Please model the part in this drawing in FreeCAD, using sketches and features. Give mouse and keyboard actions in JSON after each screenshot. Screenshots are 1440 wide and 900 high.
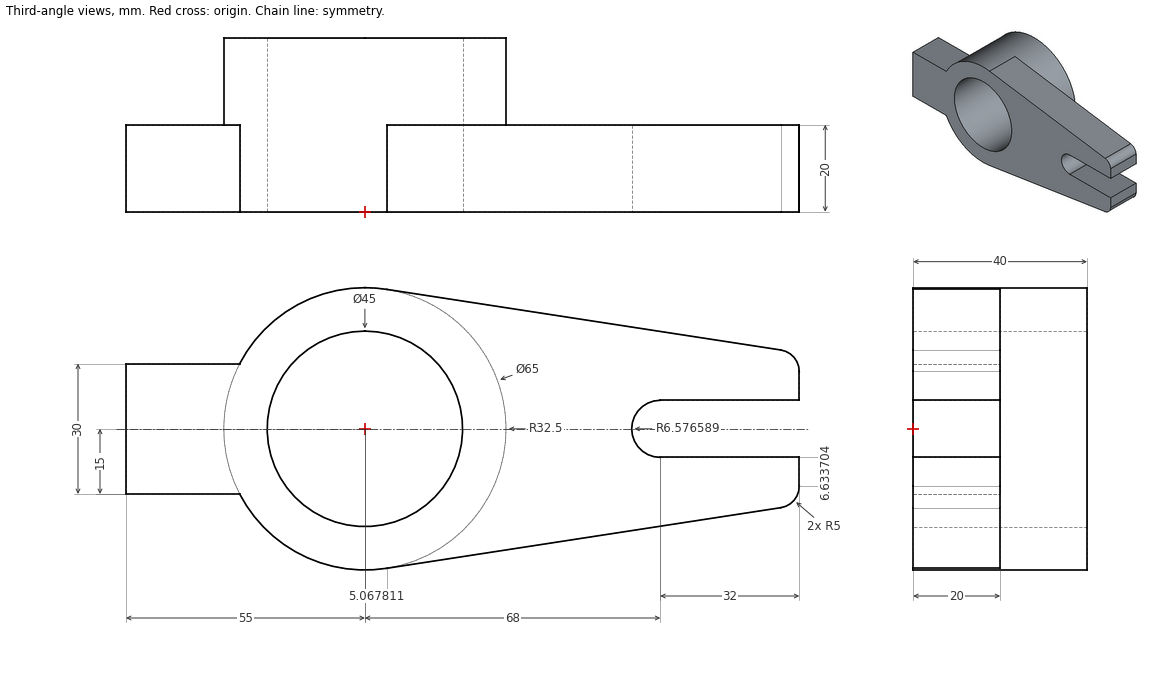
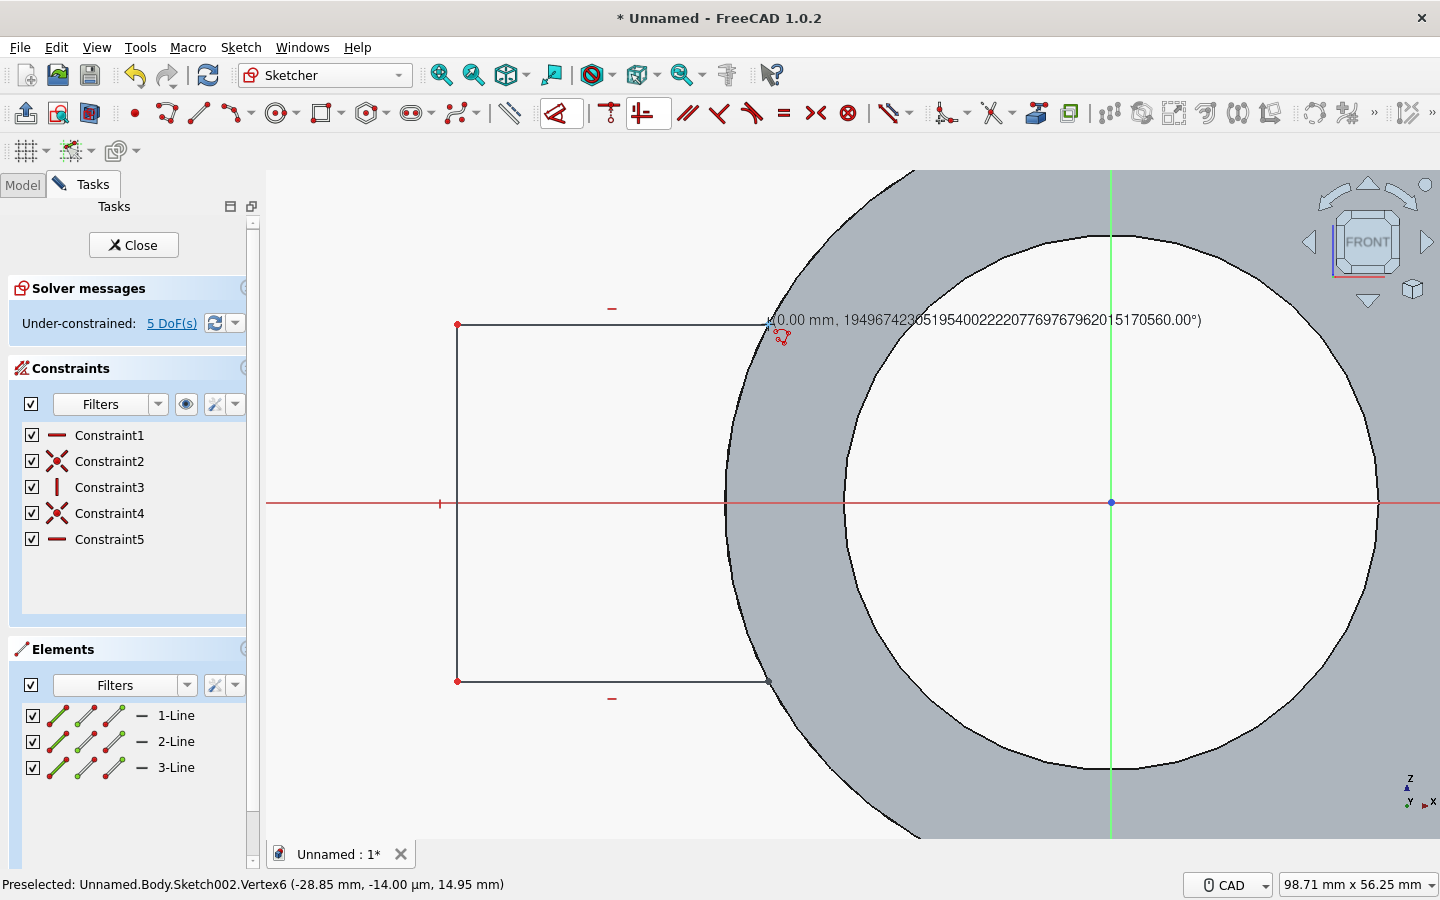
{"action": "key", "text": "g 3 a"}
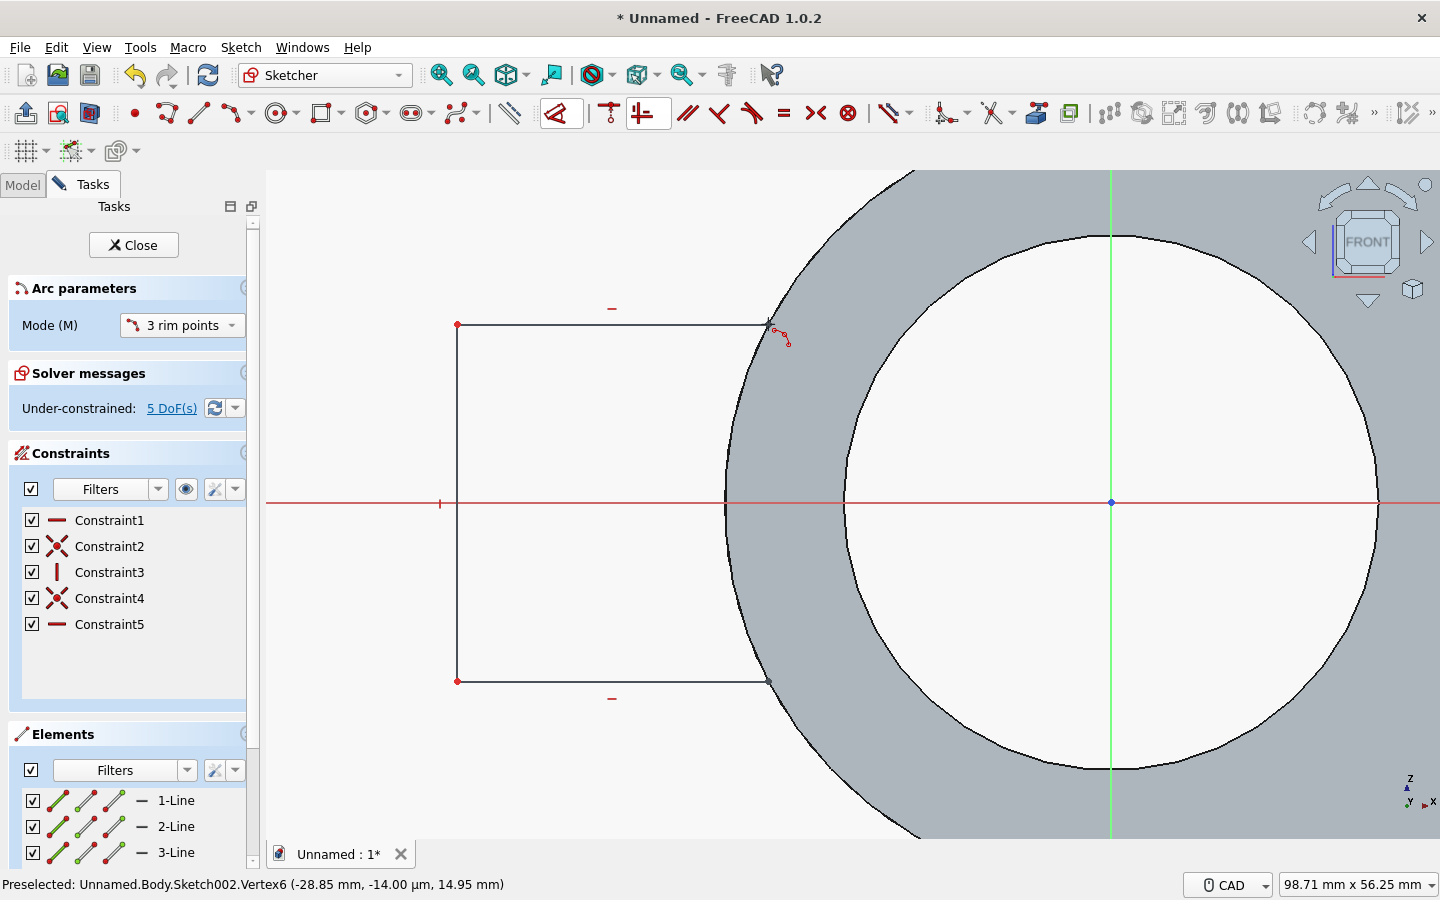
{"action": "left_click", "coordinate": [768, 325]}
{"action": "left_click", "coordinate": [768, 682]}
{"action": "left_click", "coordinate": [726, 466]}
{"action": "key", "text": "Escape"}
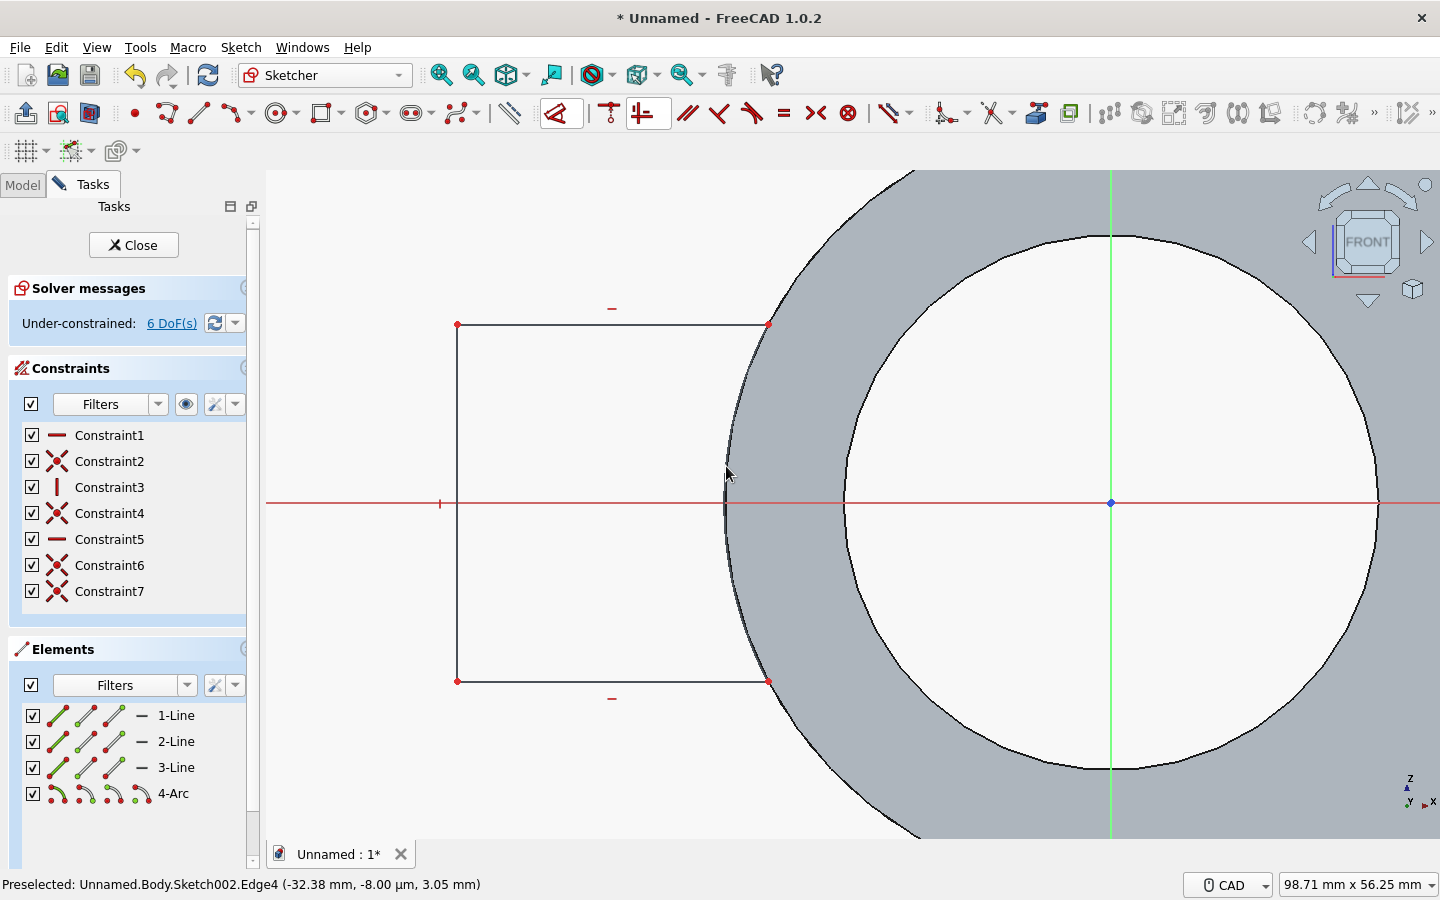
{"action": "left_click_drag", "start_coordinate": [1100, 493], "coordinate": [1121, 514]}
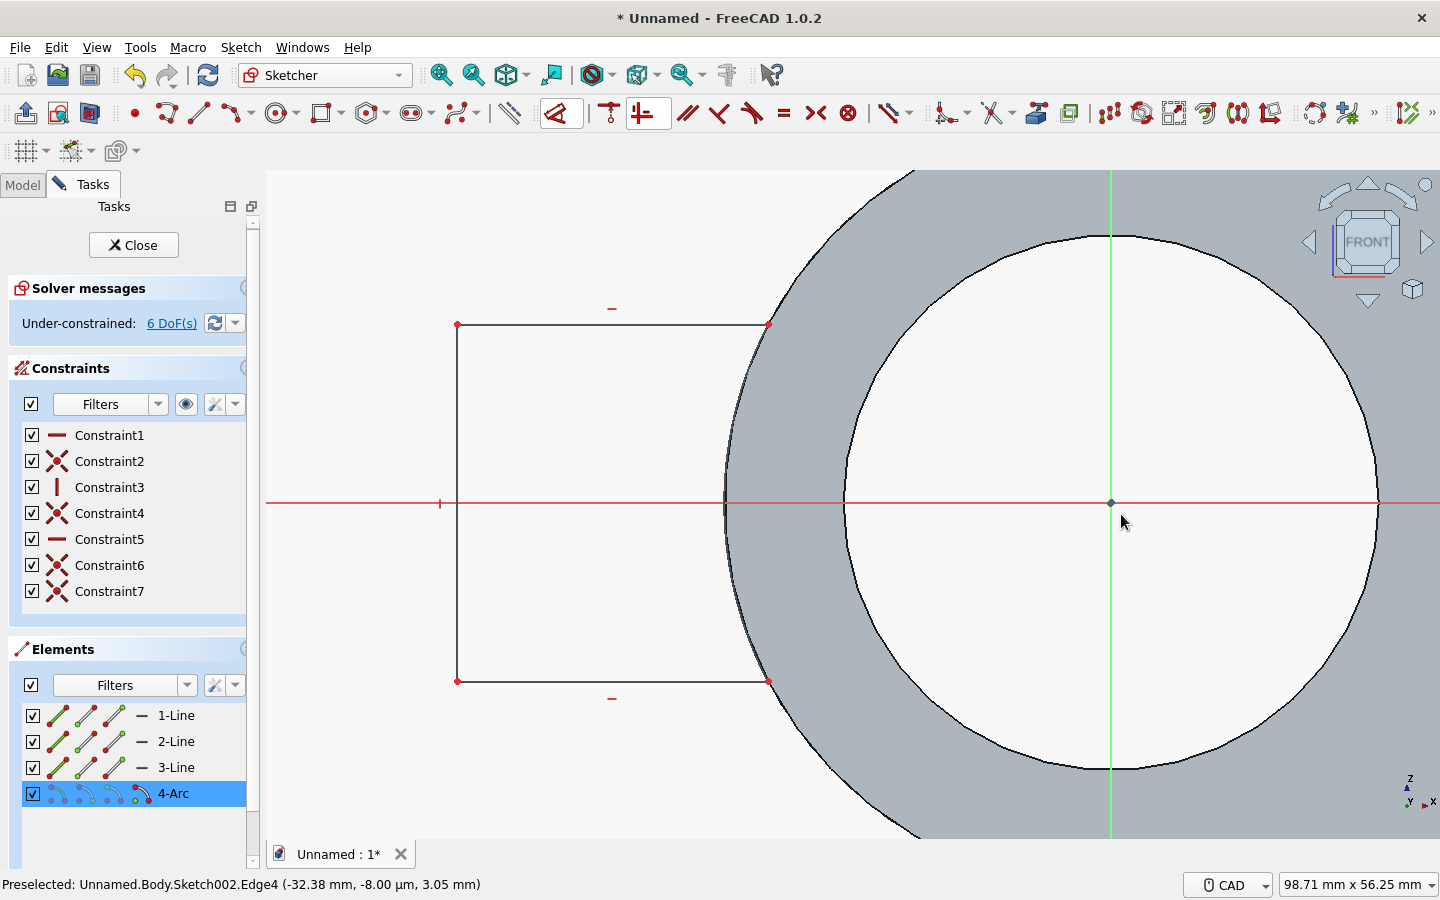
{"action": "left_click", "coordinate": [610, 114]}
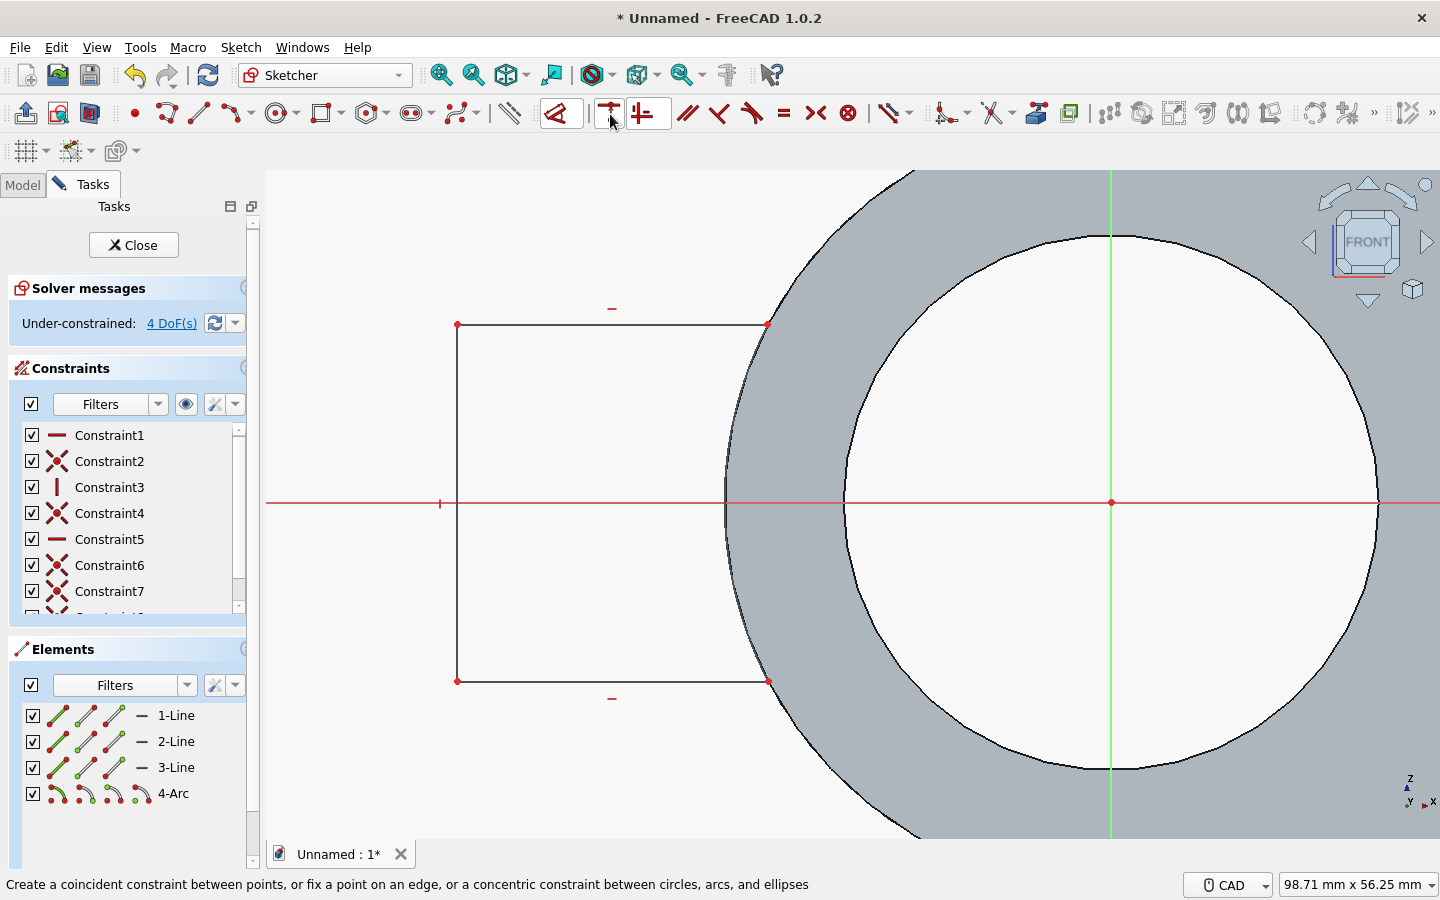
{"action": "left_click", "coordinate": [556, 114]}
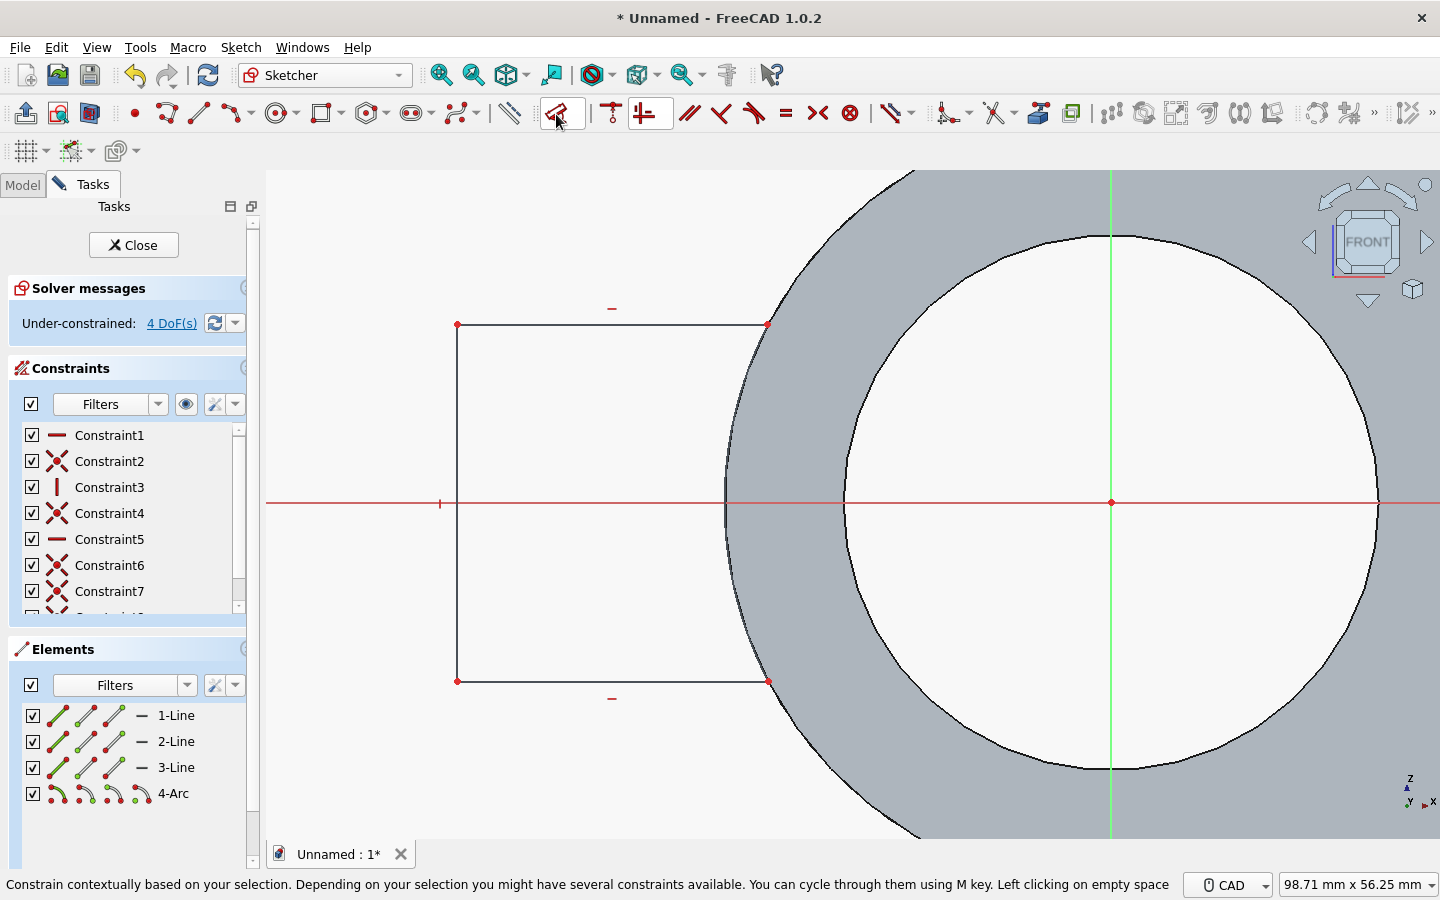
{"action": "left_click", "coordinate": [732, 430]}
{"action": "left_click", "coordinate": [701, 424]}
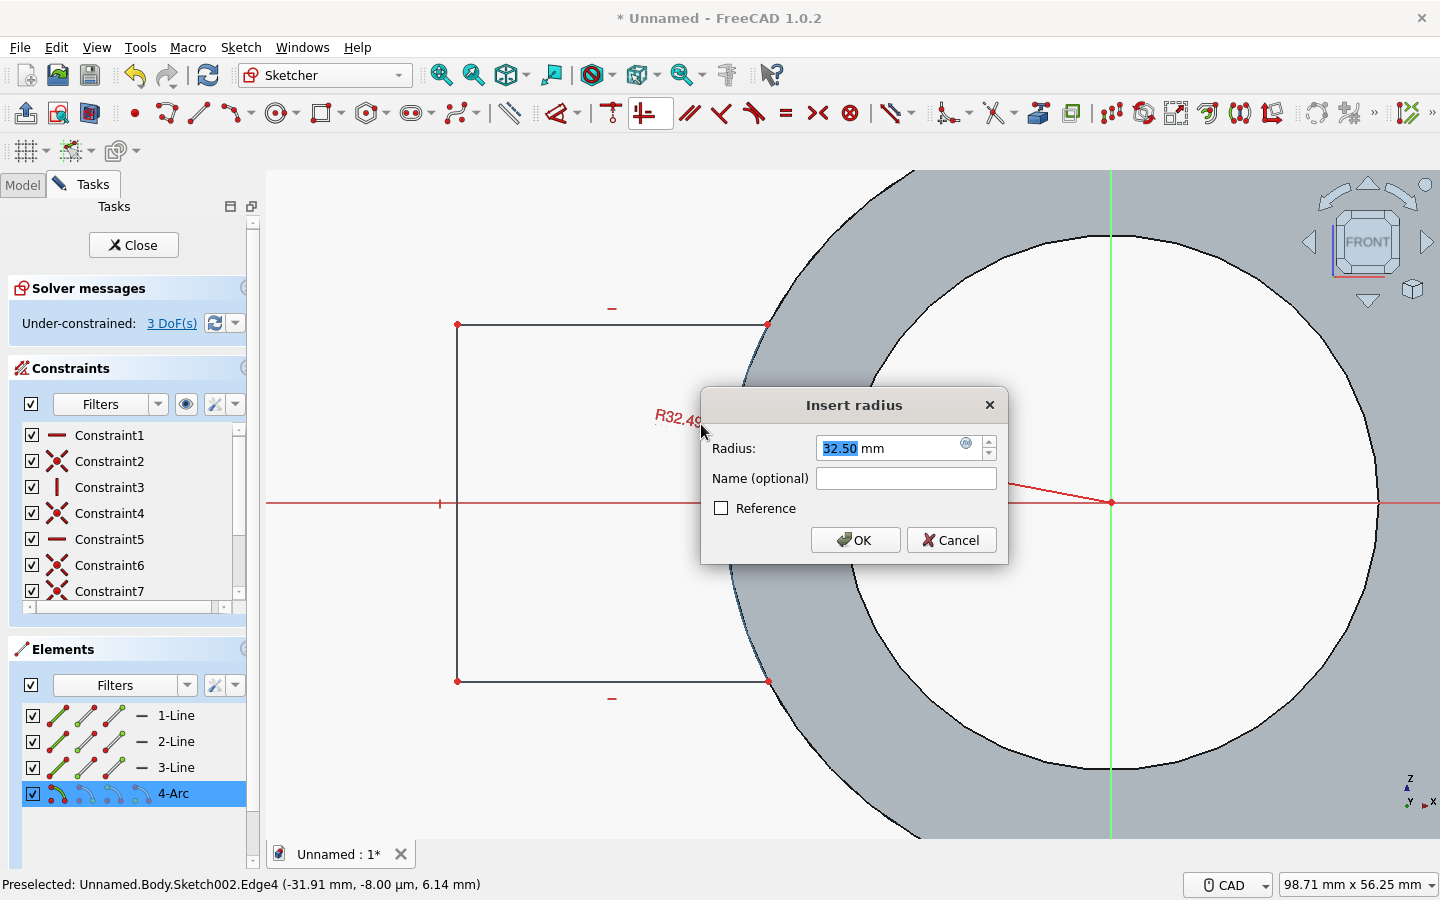
{"action": "type", "text": "32.5"}
{"action": "key", "text": "Return"}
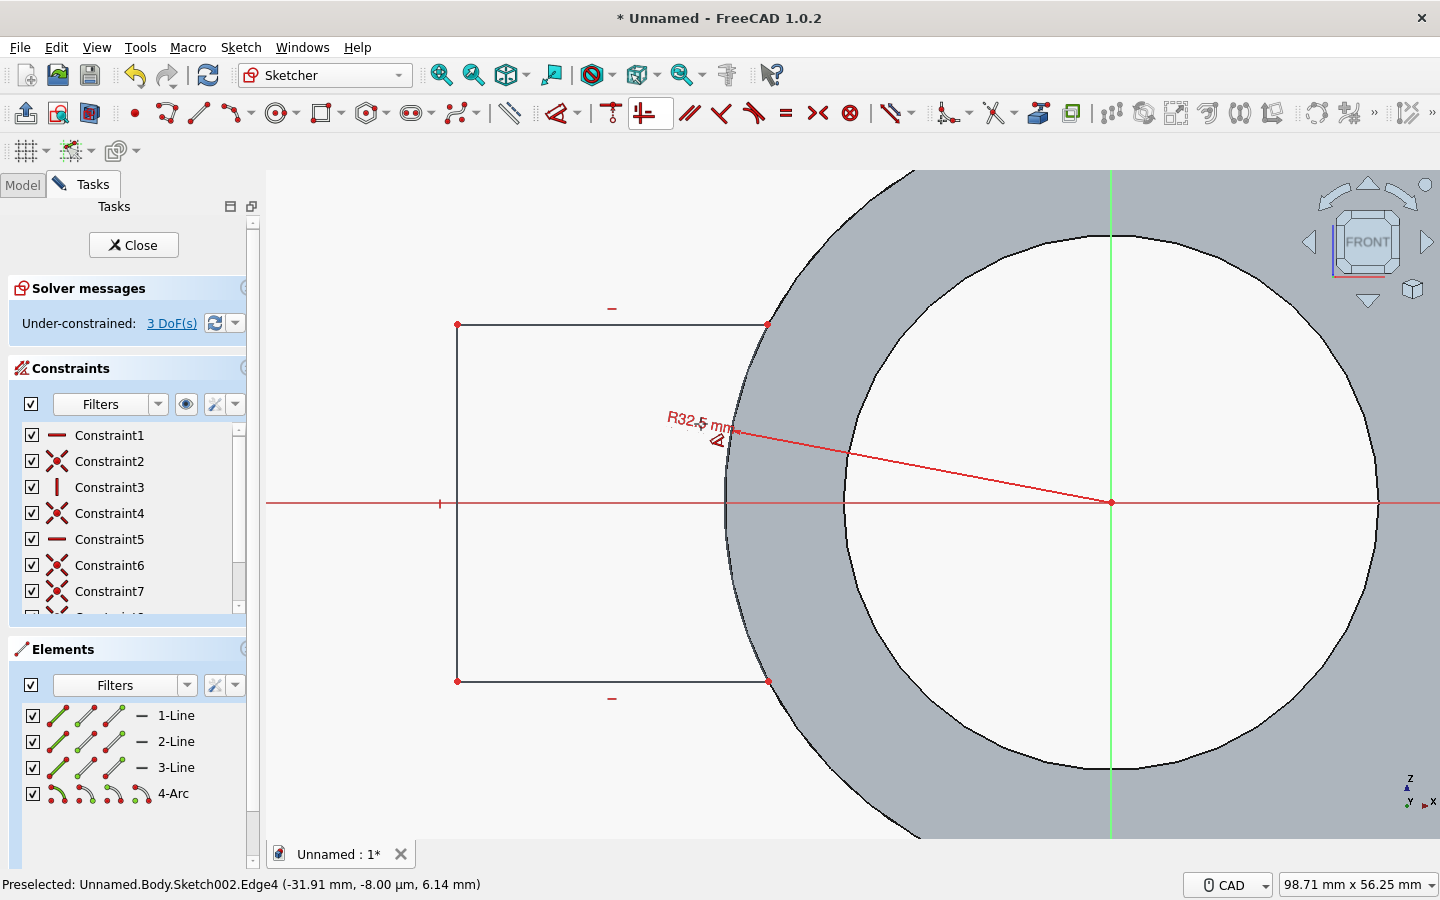
{"action": "left_click", "coordinate": [457, 575]}
{"action": "left_click", "coordinate": [423, 421]}